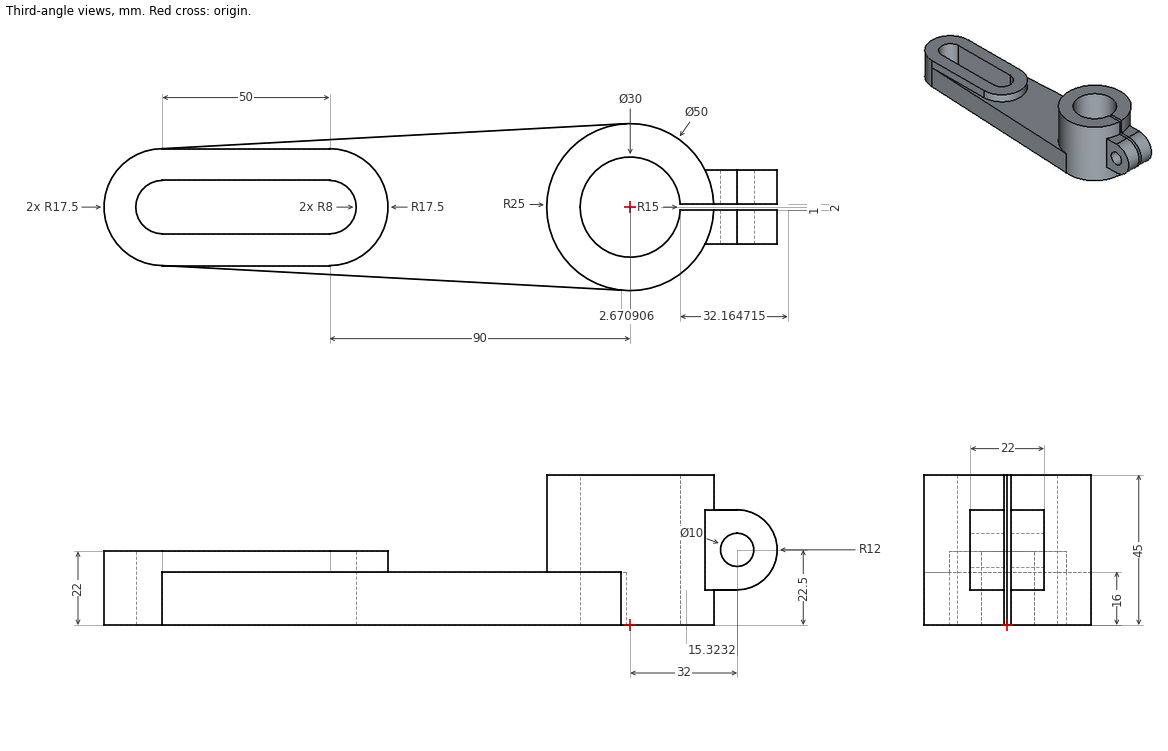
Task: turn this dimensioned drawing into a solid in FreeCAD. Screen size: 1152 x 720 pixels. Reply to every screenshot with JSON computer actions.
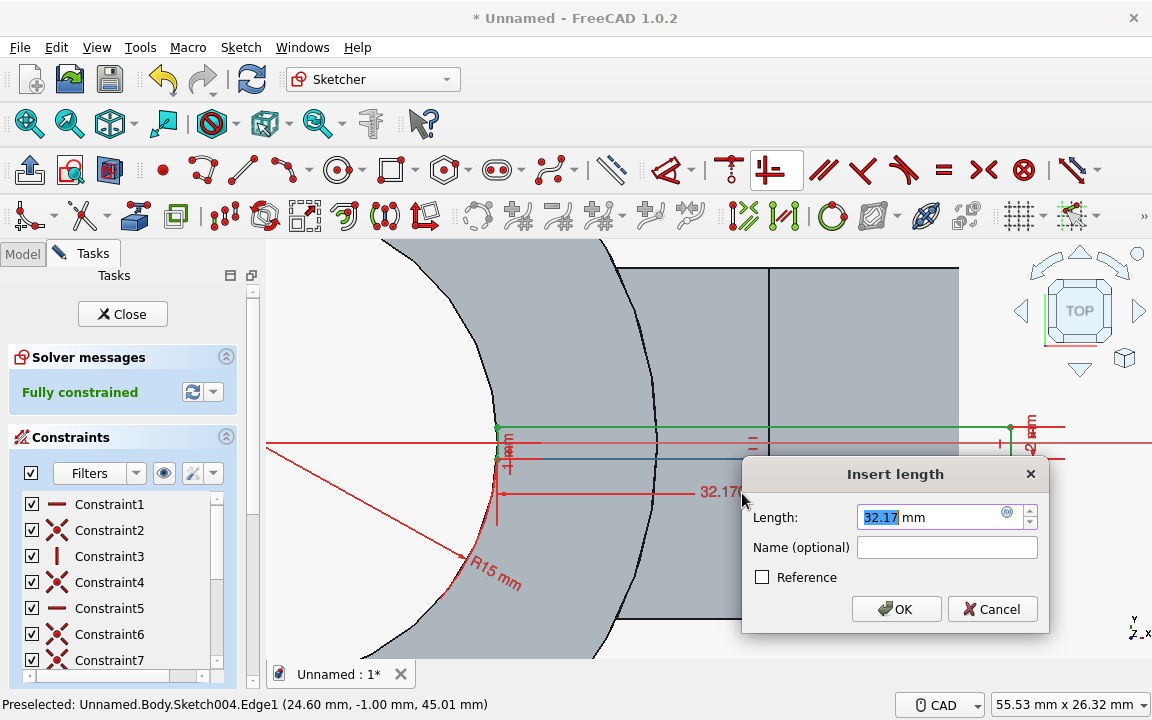
{"action": "type", "text": "32.164715"}
{"action": "key", "text": "Return"}
{"action": "key", "text": "Escape"}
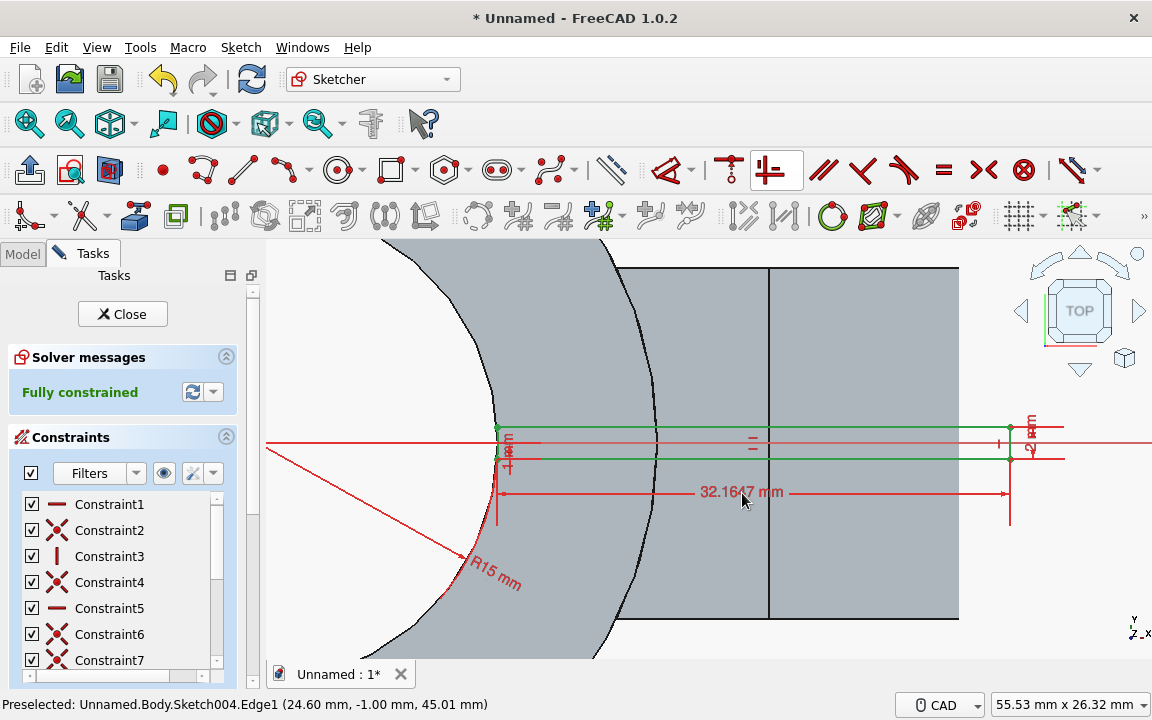
{"action": "left_click", "coordinate": [123, 314]}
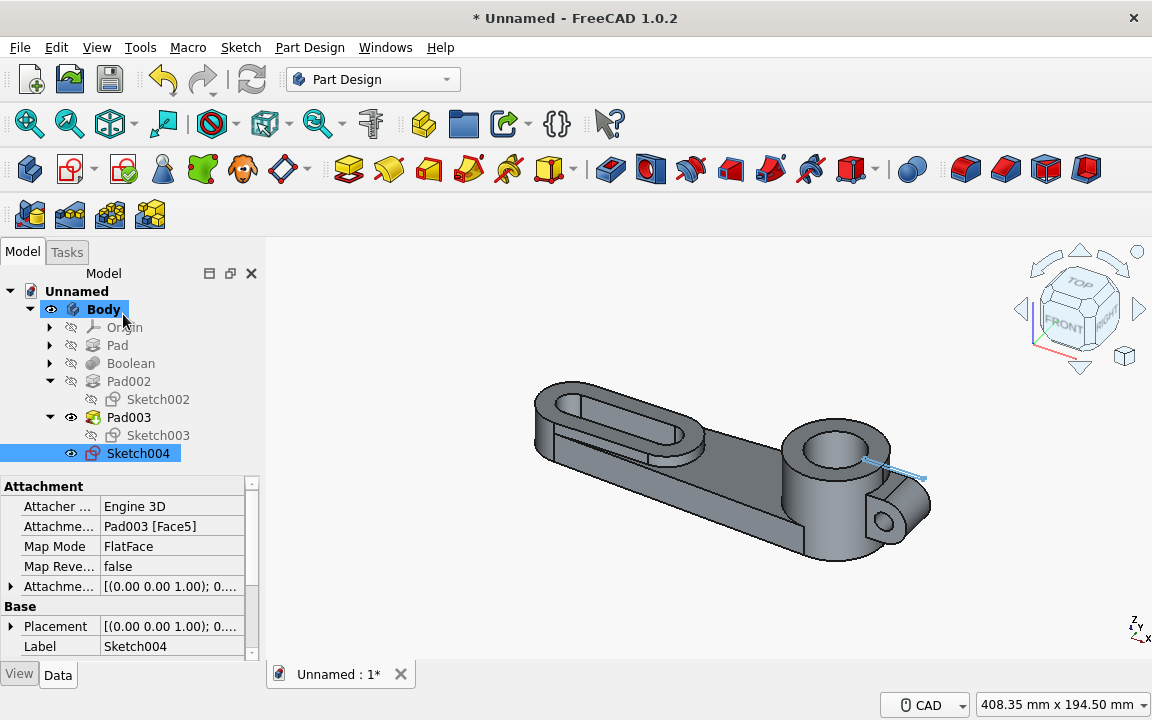
{"action": "left_click", "coordinate": [612, 170]}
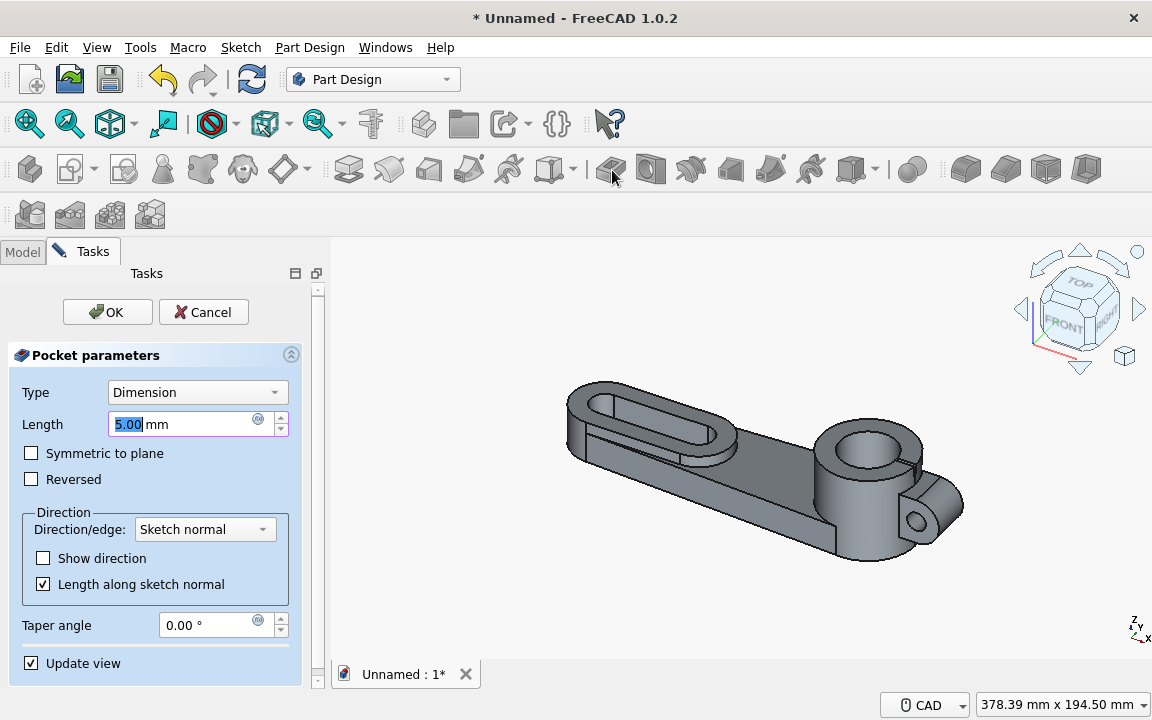
{"action": "left_click", "coordinate": [198, 392]}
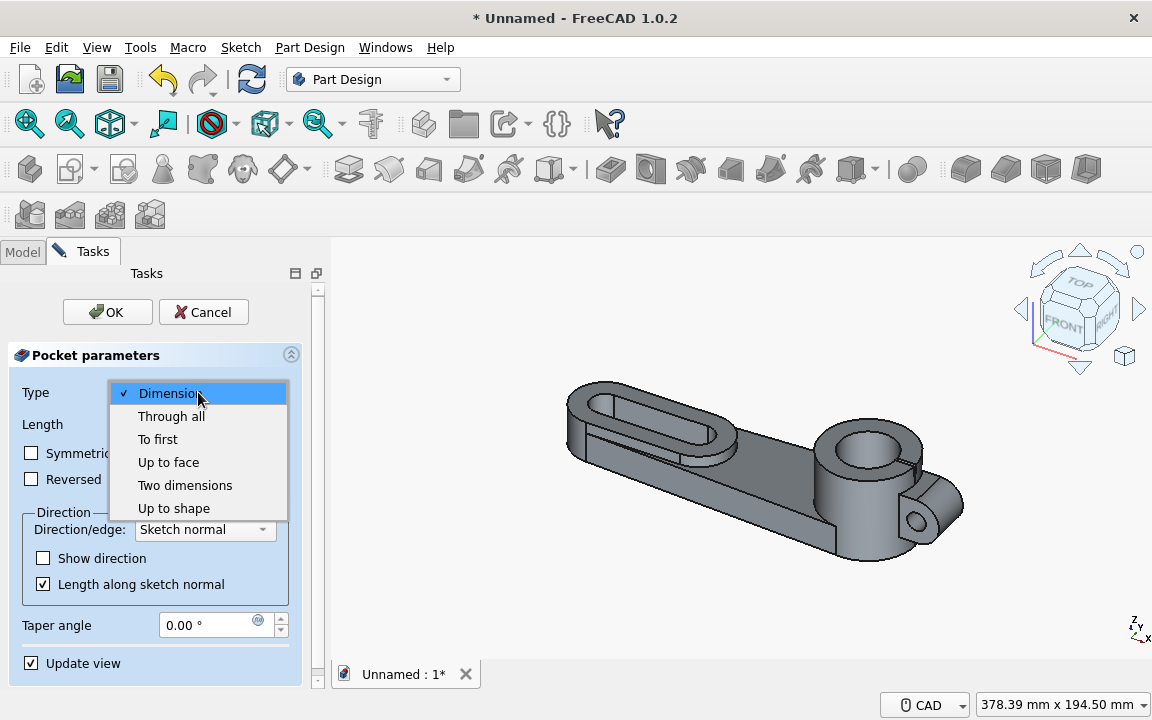
{"action": "left_click", "coordinate": [198, 416]}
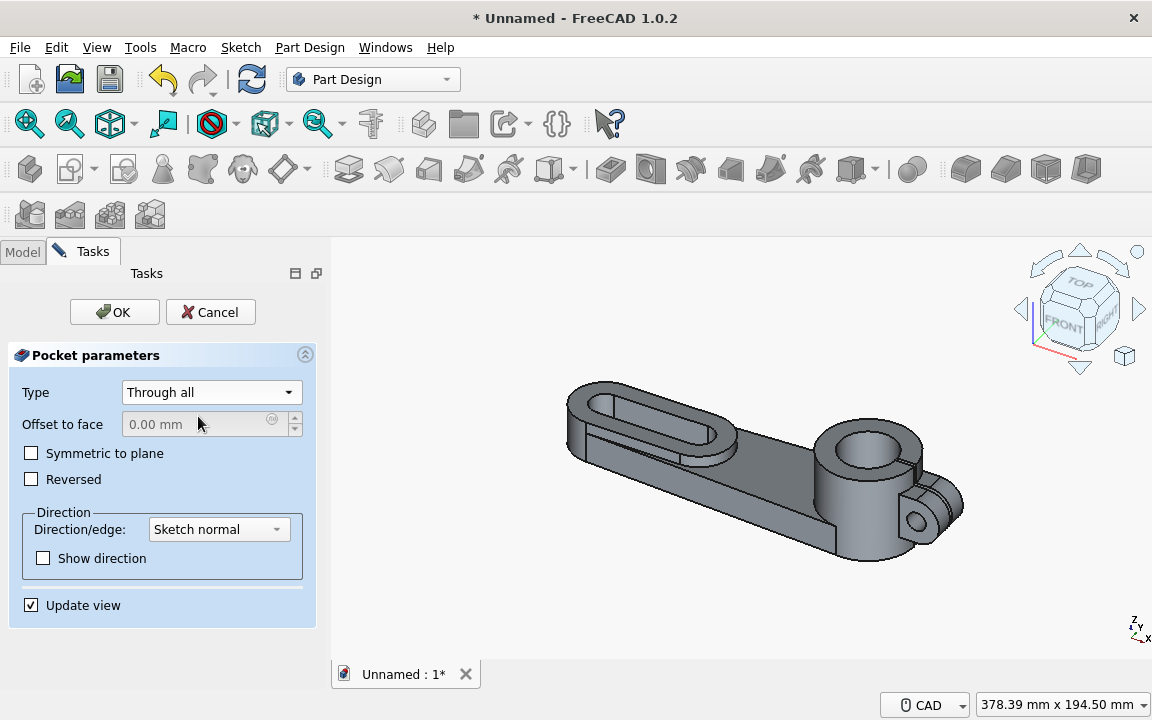
{"action": "left_click", "coordinate": [115, 312]}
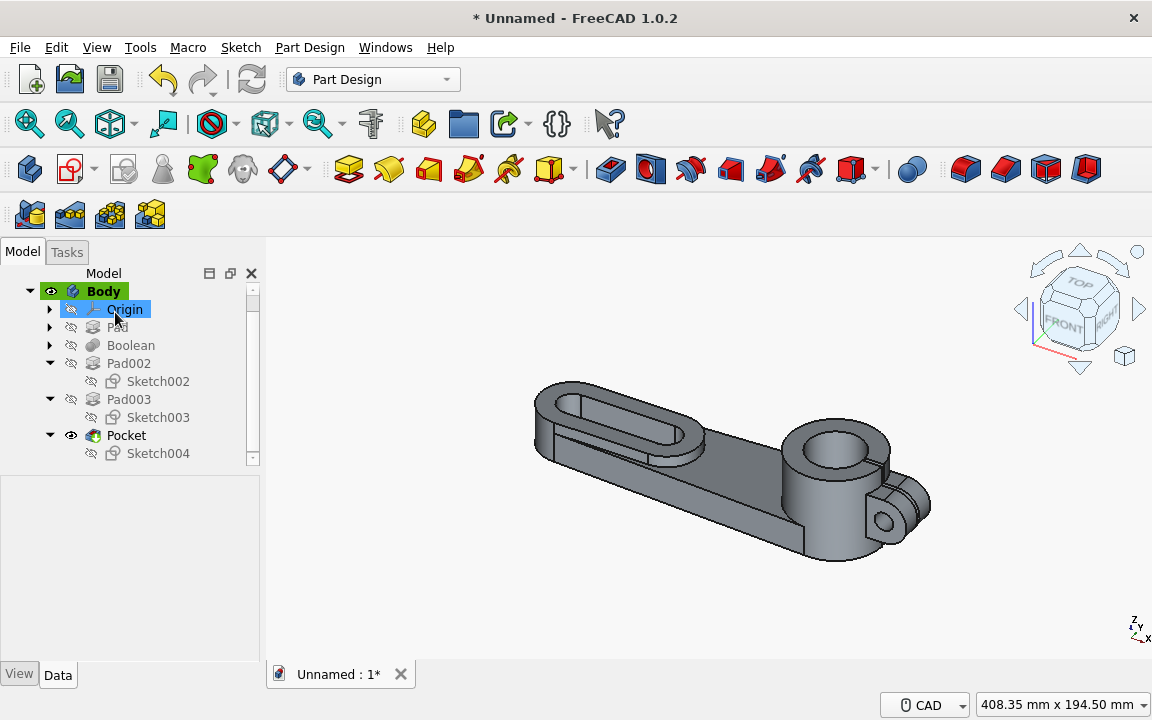
{"action": "key", "text": "0"}